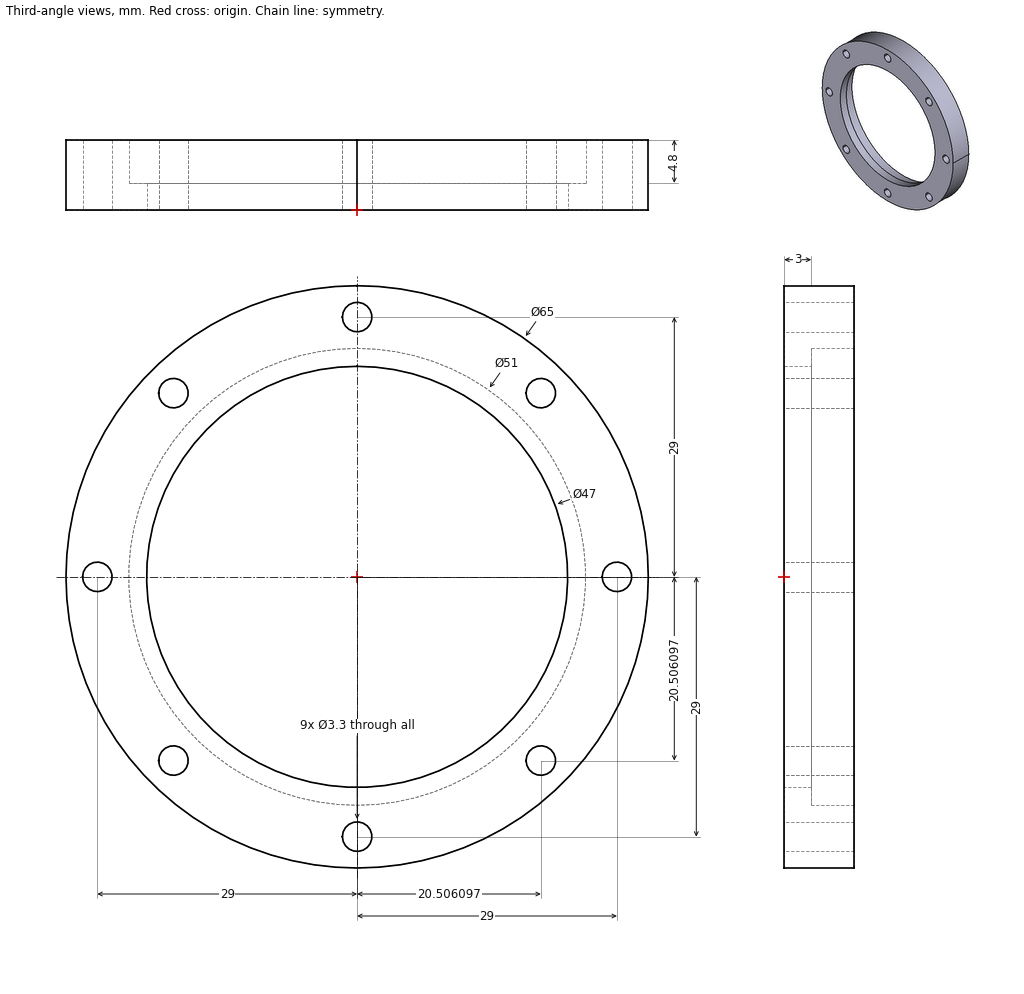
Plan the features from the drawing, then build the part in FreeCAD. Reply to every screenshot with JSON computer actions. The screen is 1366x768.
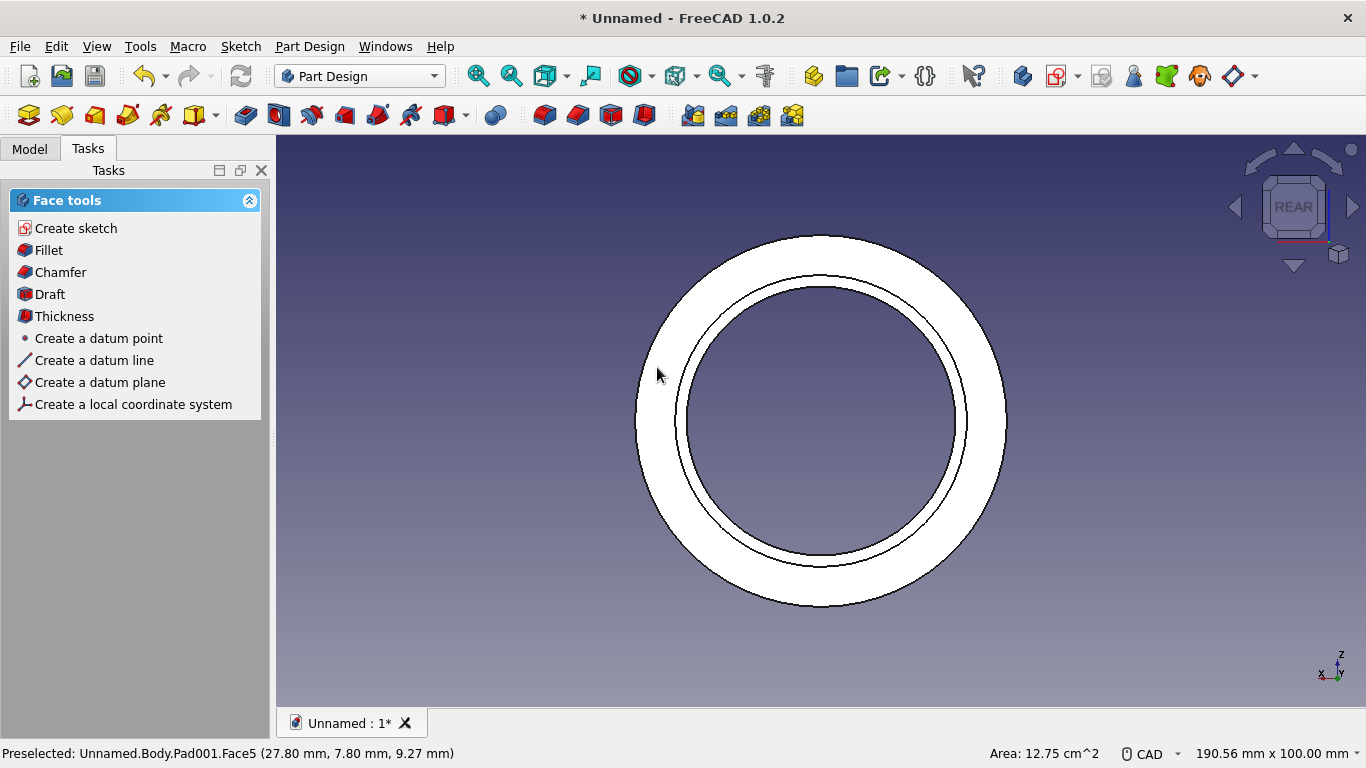
{"action": "left_click", "coordinate": [1056, 76]}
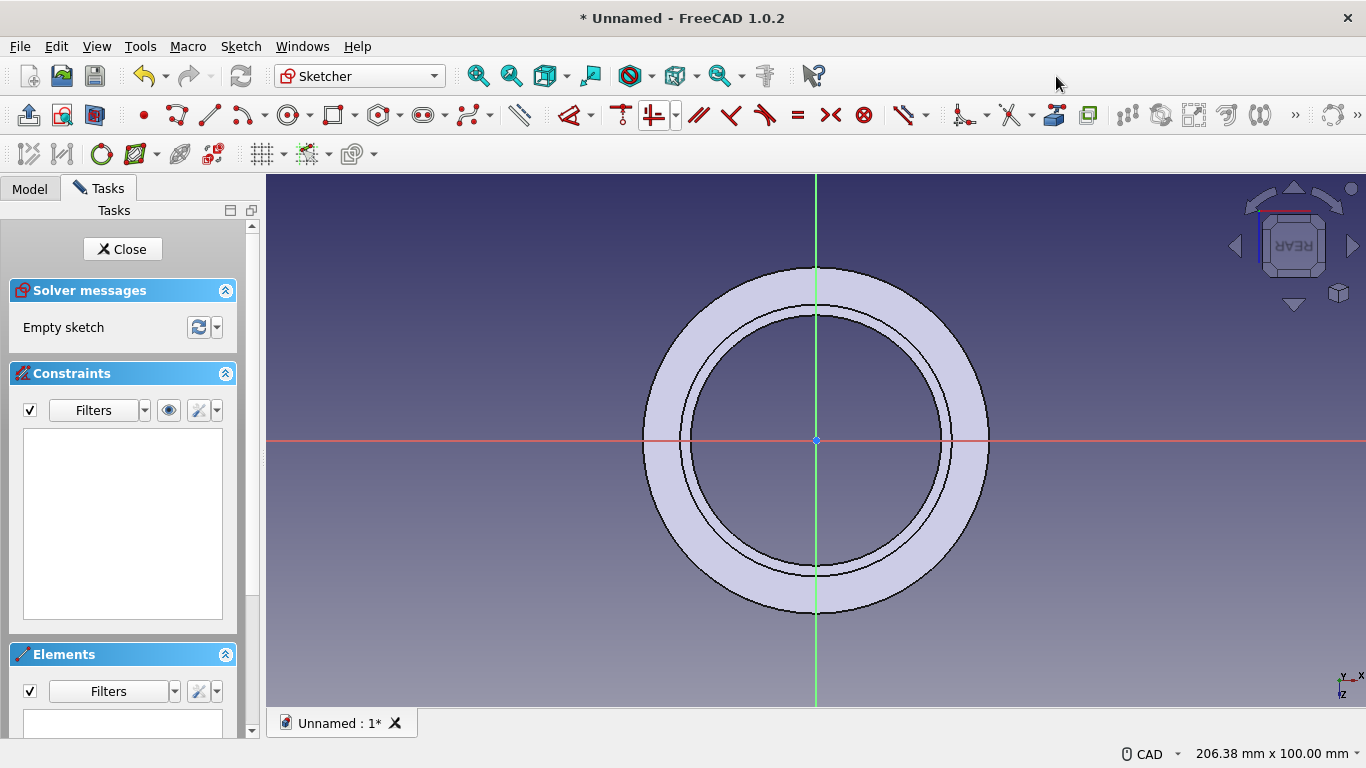
{"action": "left_click", "coordinate": [288, 116]}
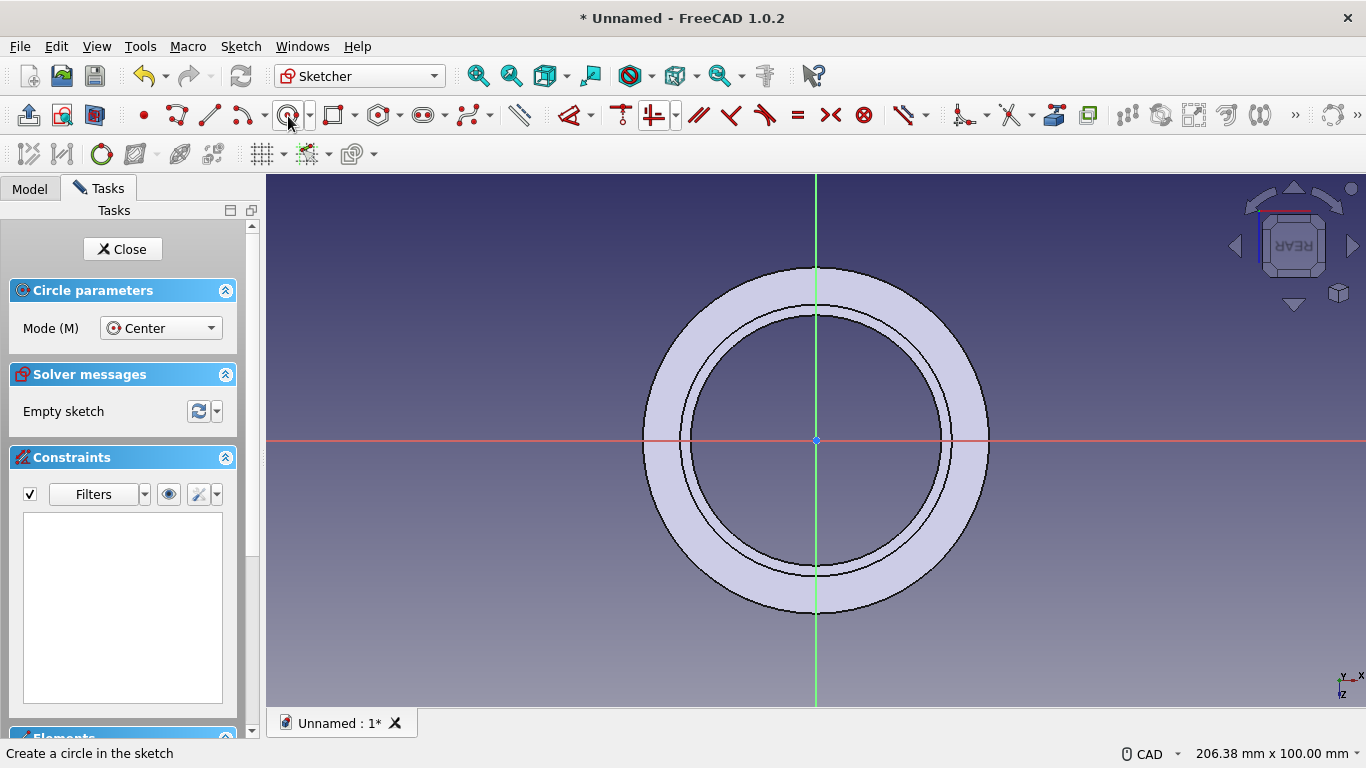
{"action": "scroll", "coordinate": [816, 286], "scroll_direction": "up", "scroll_amount": 5}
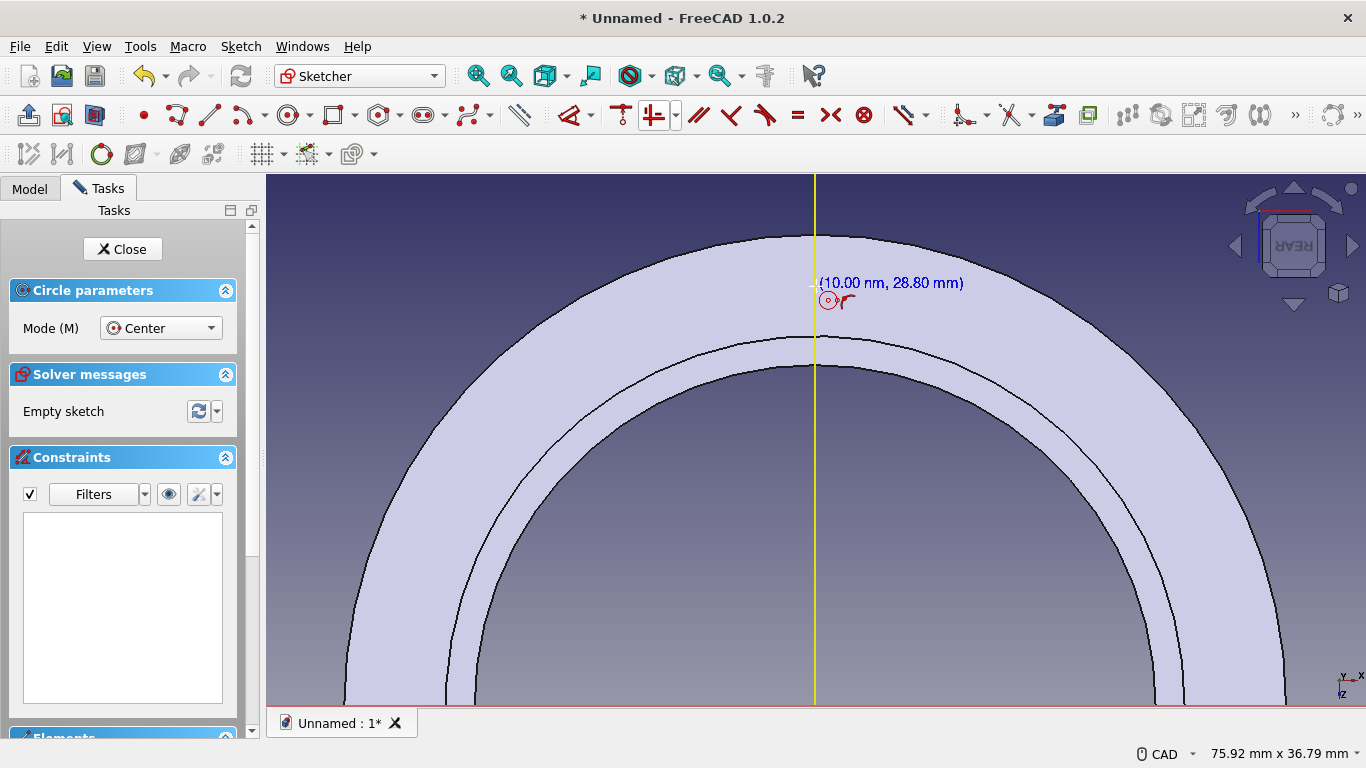
{"action": "left_click", "coordinate": [815, 285]}
{"action": "mouse_move", "coordinate": [832, 269]}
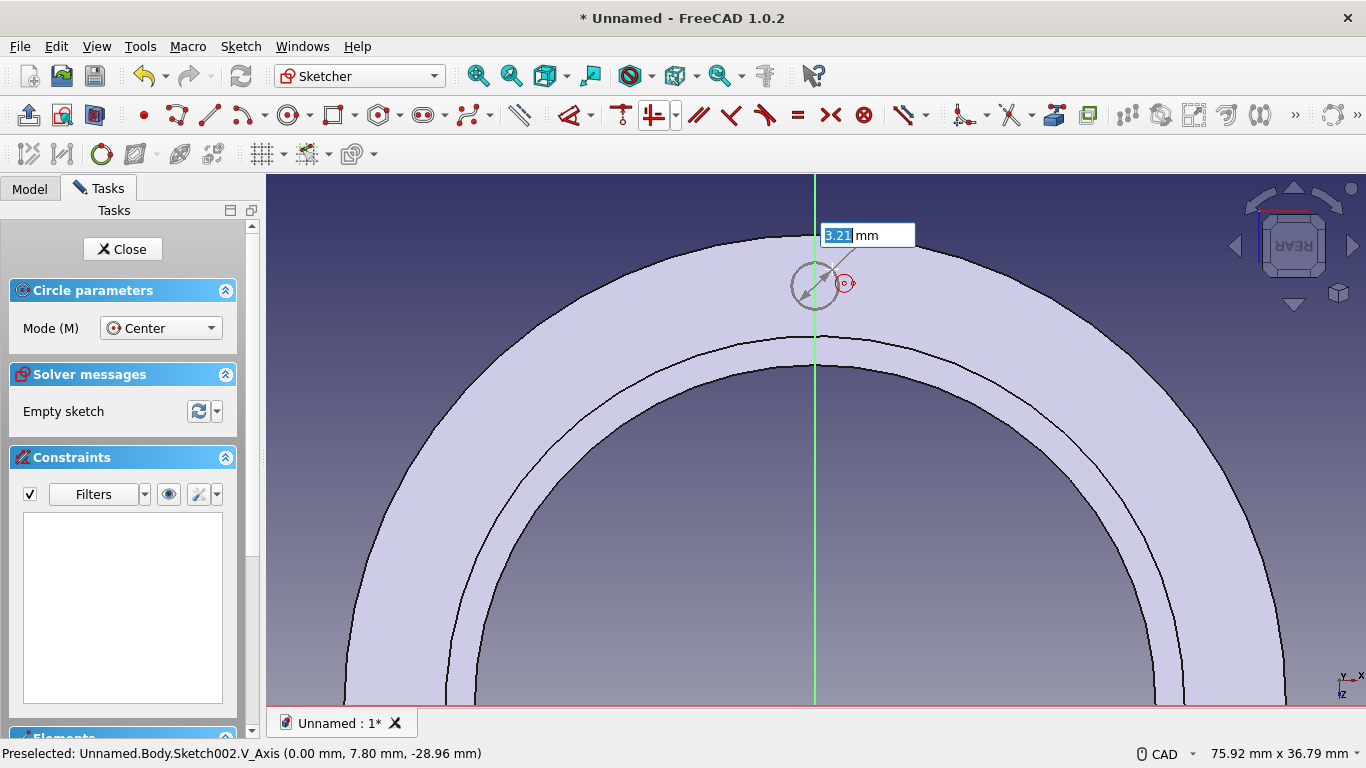
{"action": "type", "text": "3.3"}
{"action": "key", "text": "Return"}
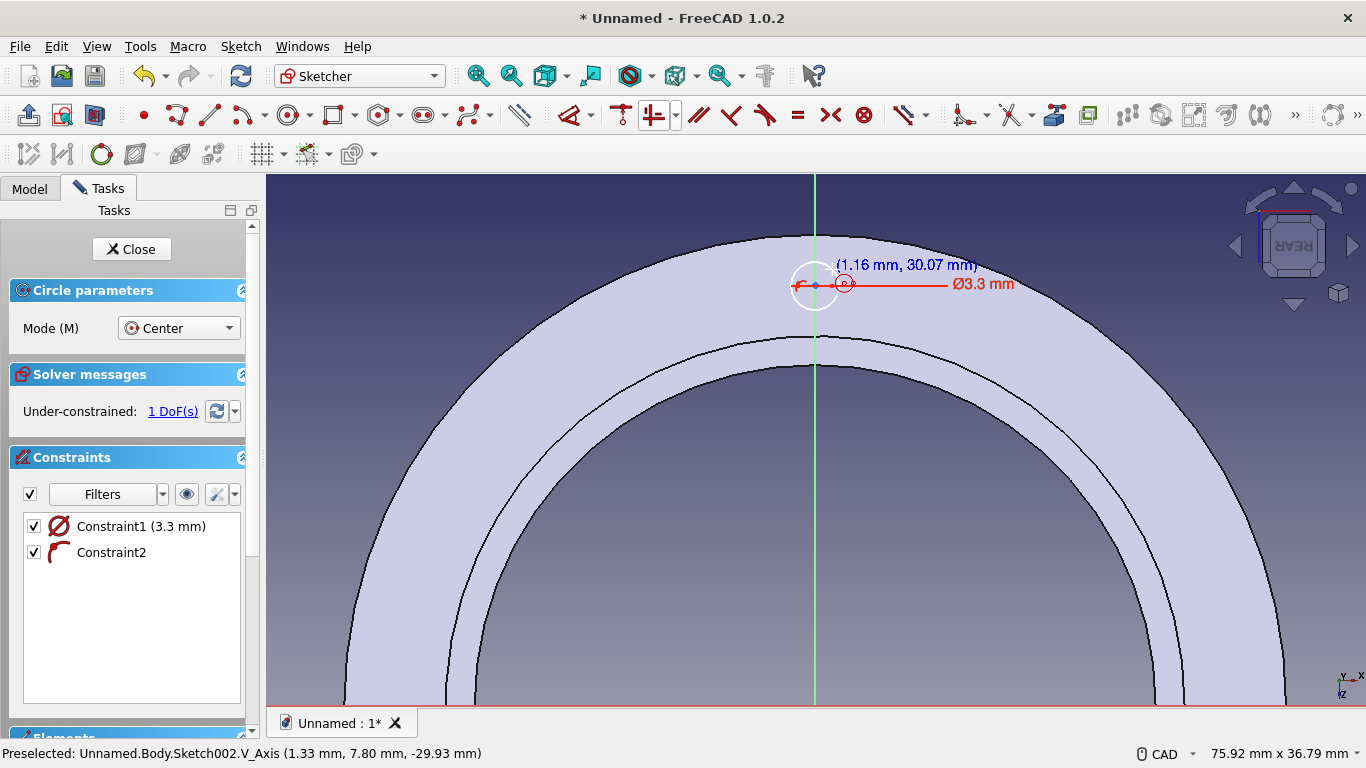
{"action": "left_click", "coordinate": [1112, 409]}
{"action": "mouse_move", "coordinate": [1129, 392]}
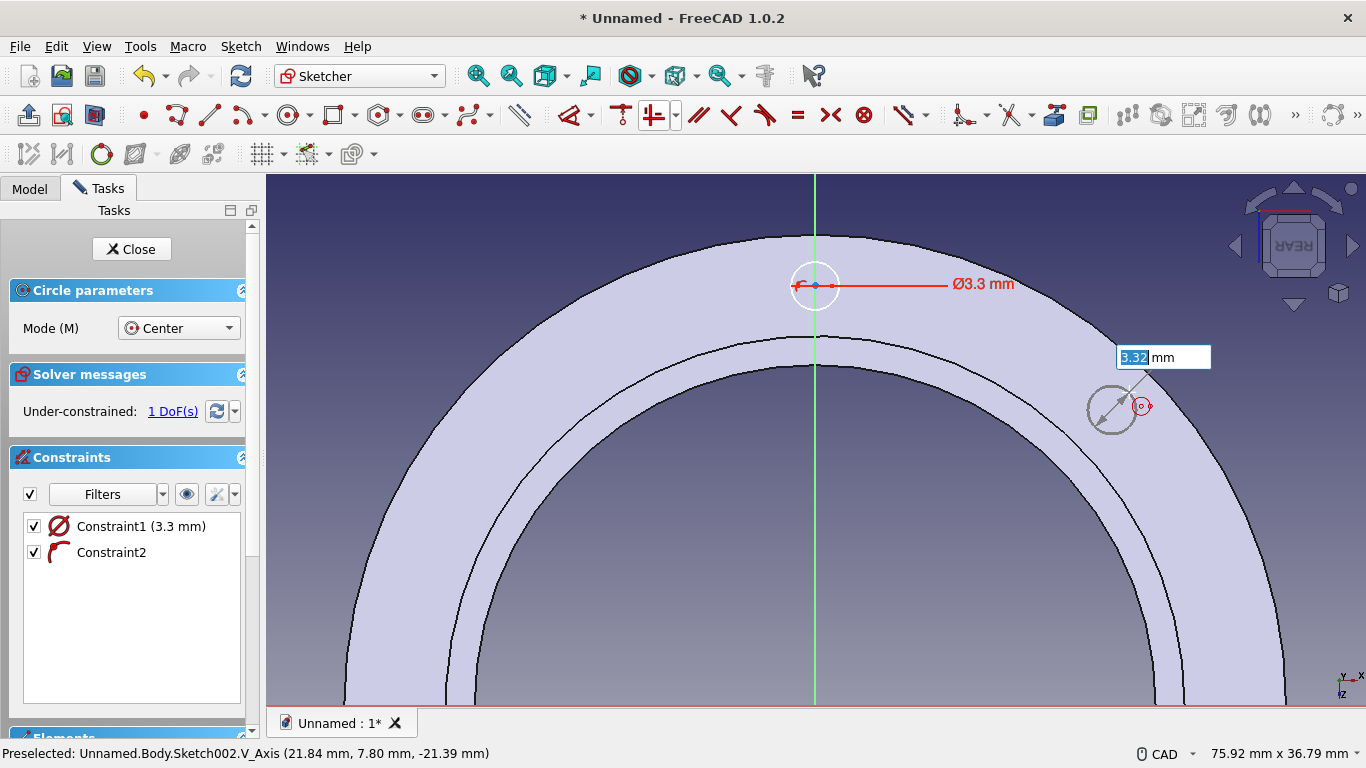
{"action": "type", "text": "3.3"}
{"action": "key", "text": "Return"}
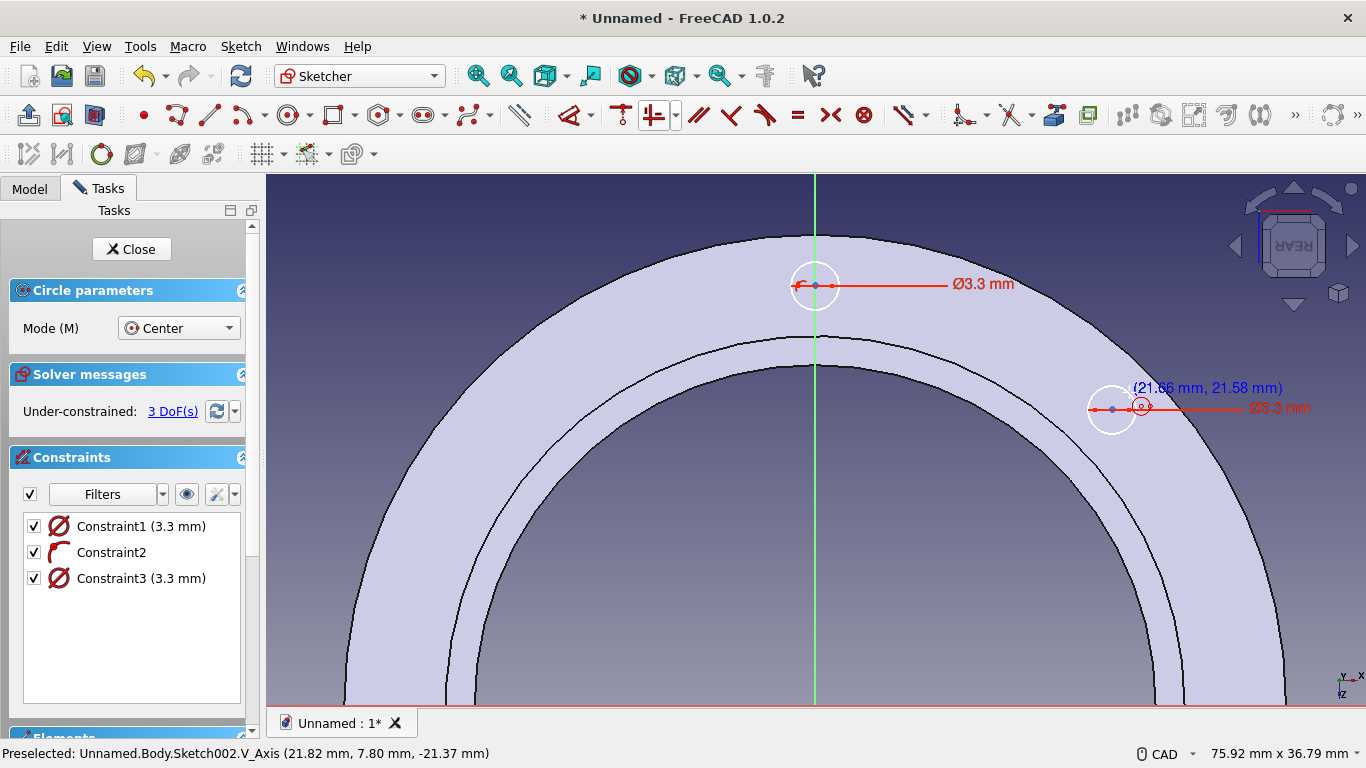
{"action": "scroll", "coordinate": [708, 286], "scroll_direction": "down", "scroll_amount": 5}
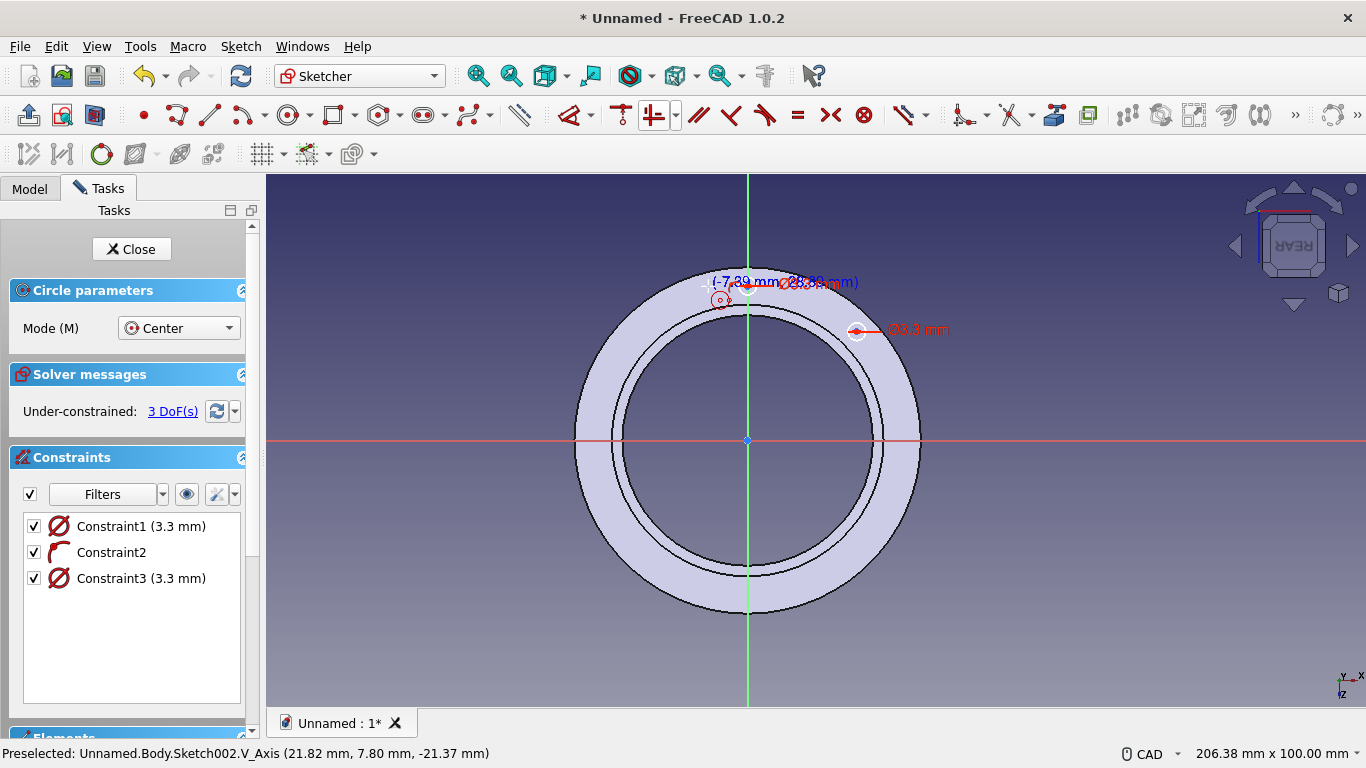
{"action": "scroll", "coordinate": [902, 440], "scroll_direction": "up", "scroll_amount": 5}